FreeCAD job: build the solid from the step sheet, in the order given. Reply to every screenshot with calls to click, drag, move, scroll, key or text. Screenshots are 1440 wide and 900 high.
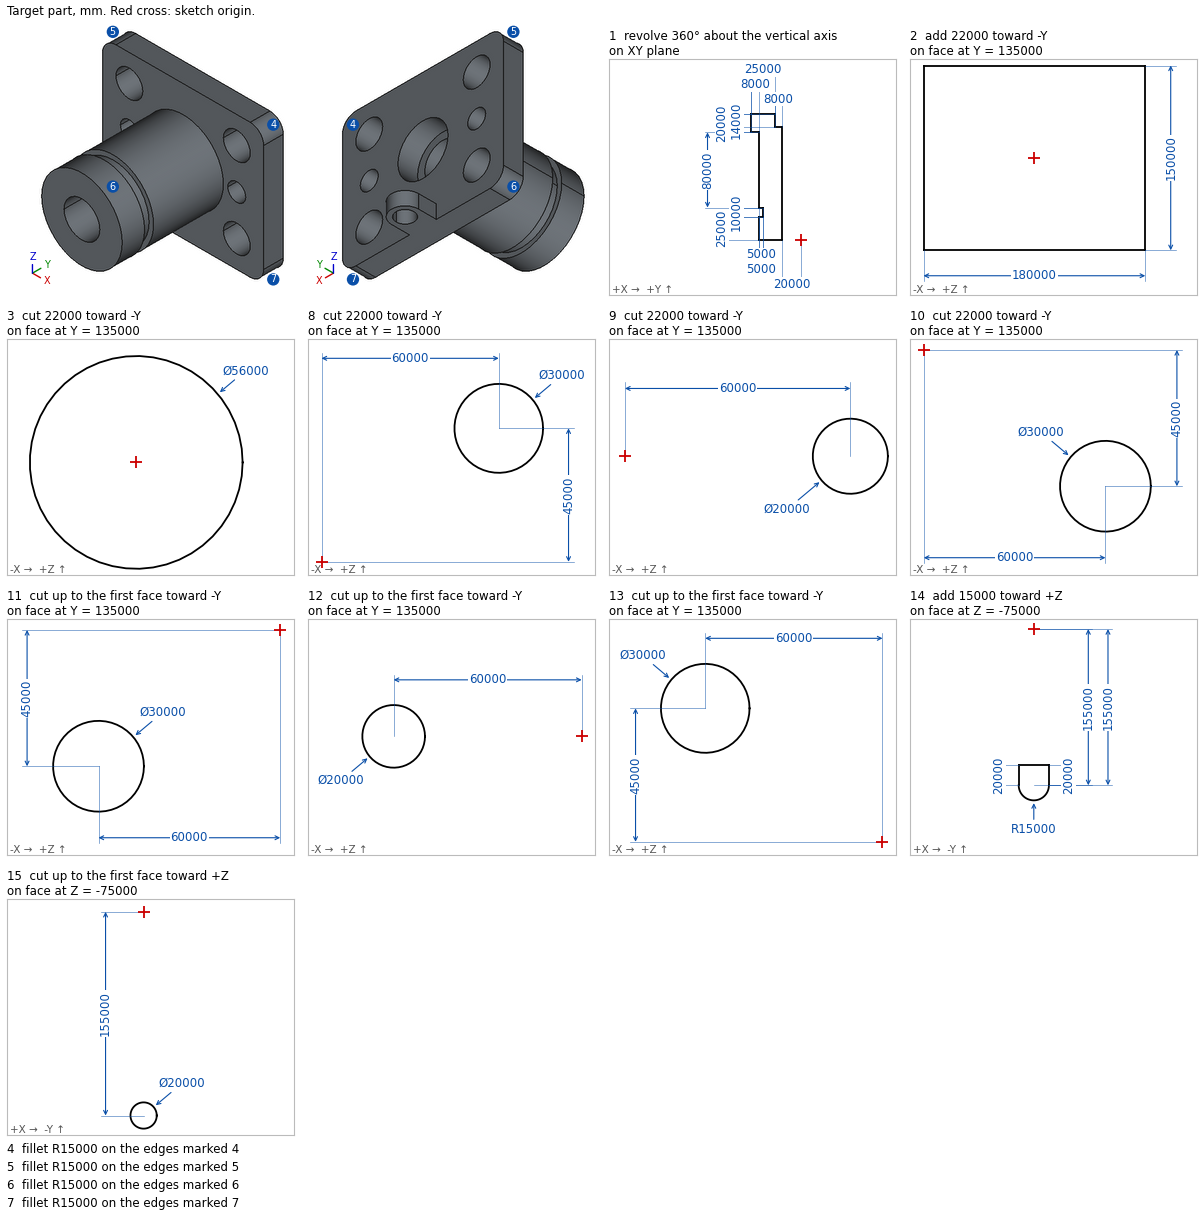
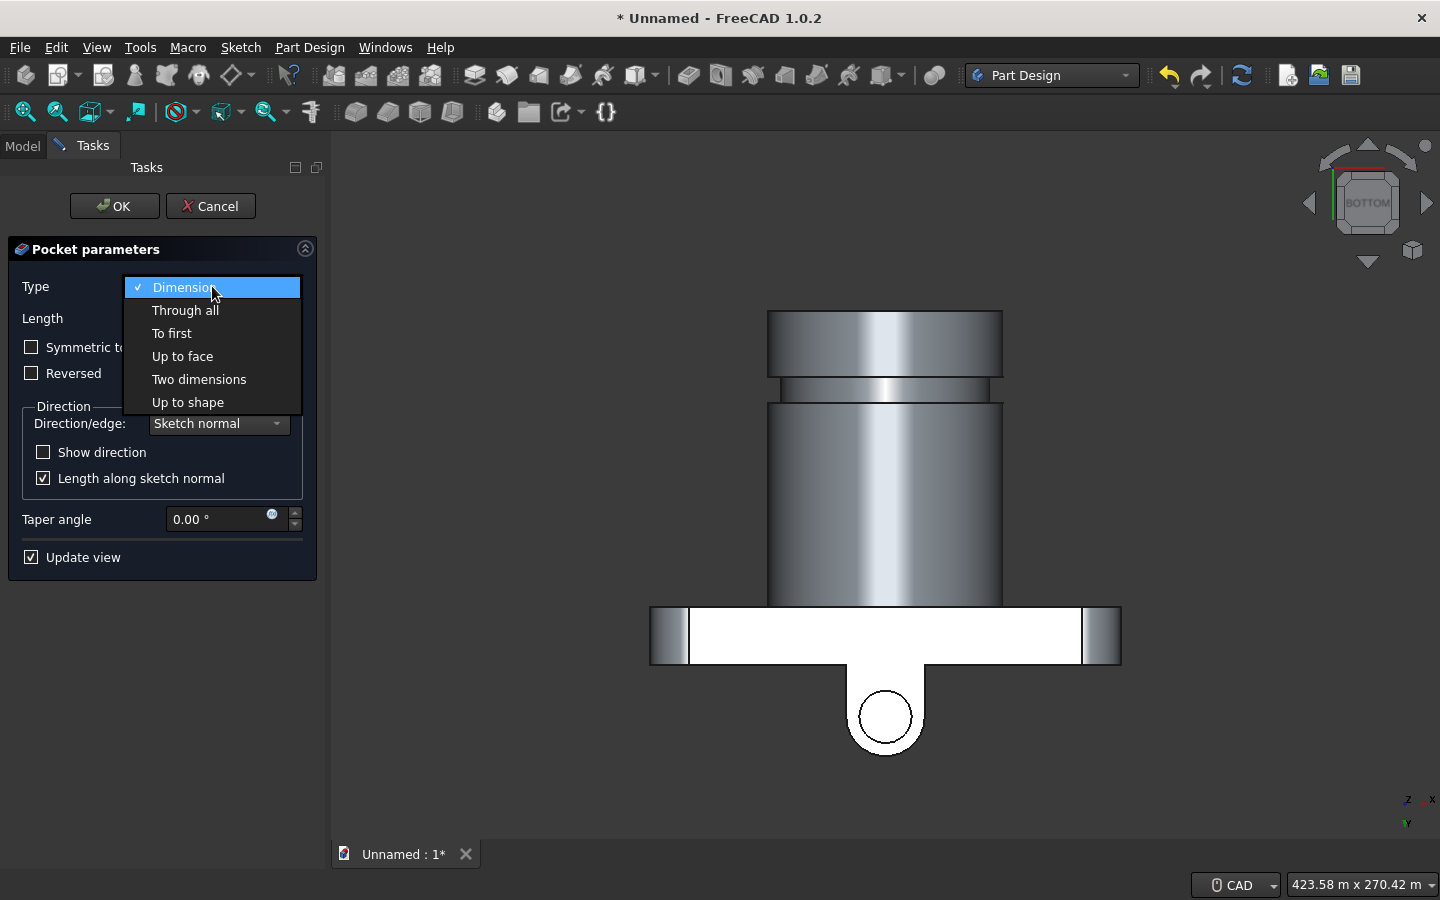
click(212, 334)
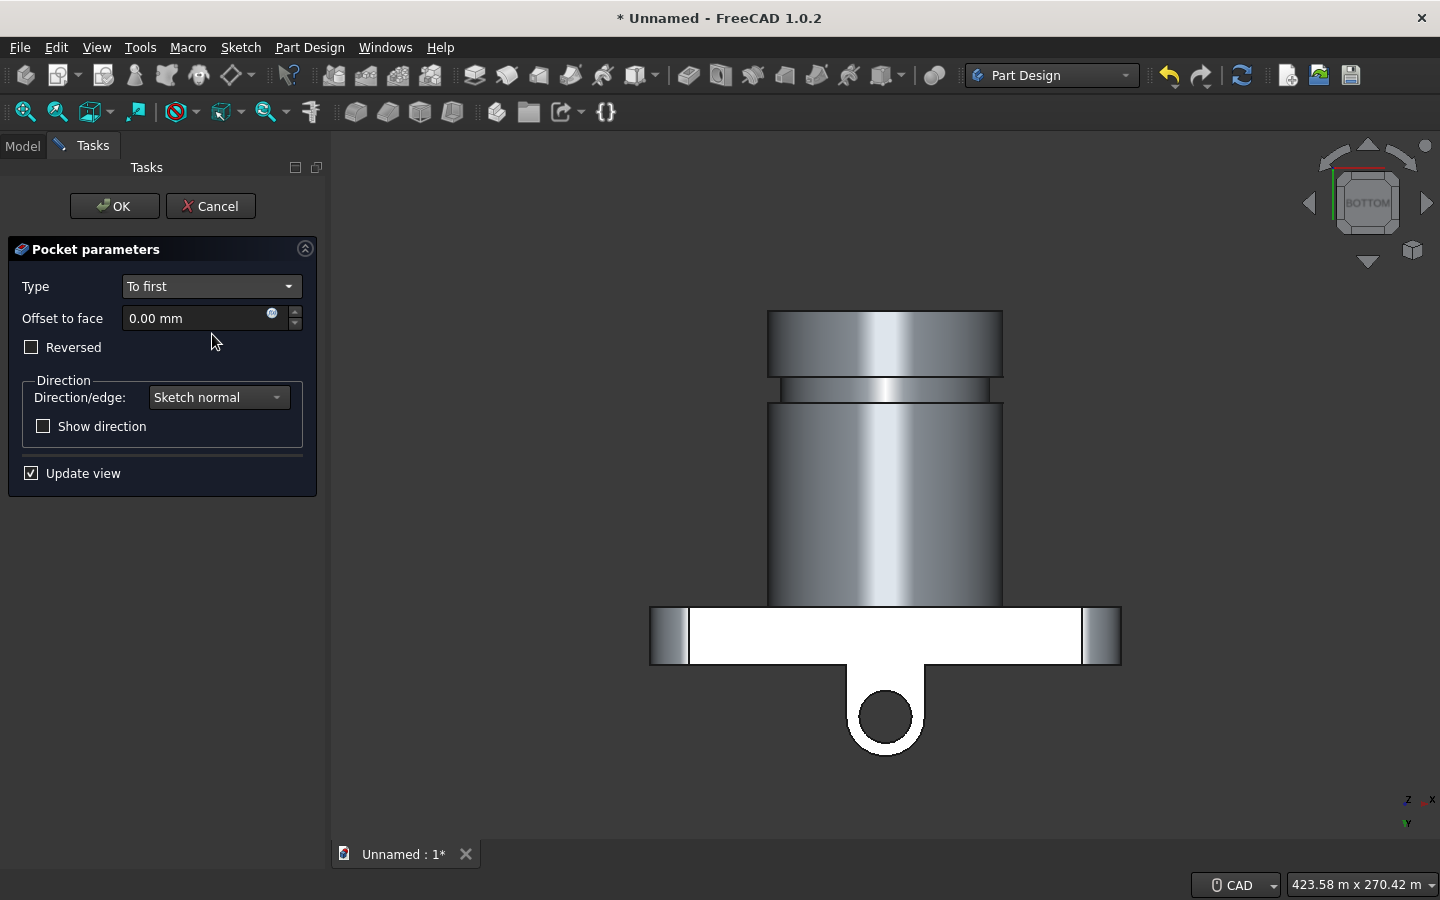
click(115, 206)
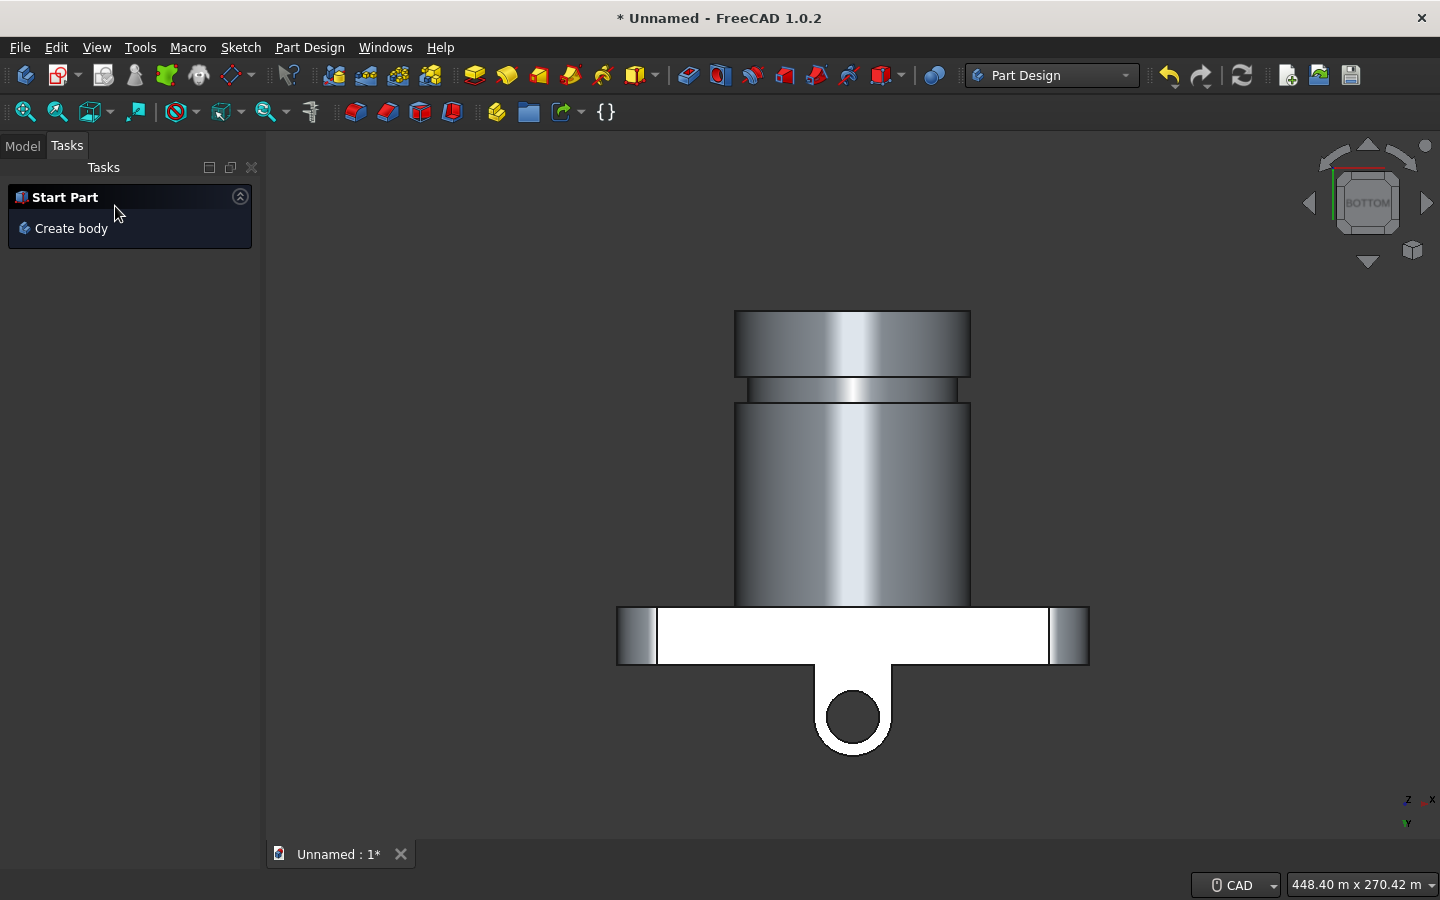
key(0)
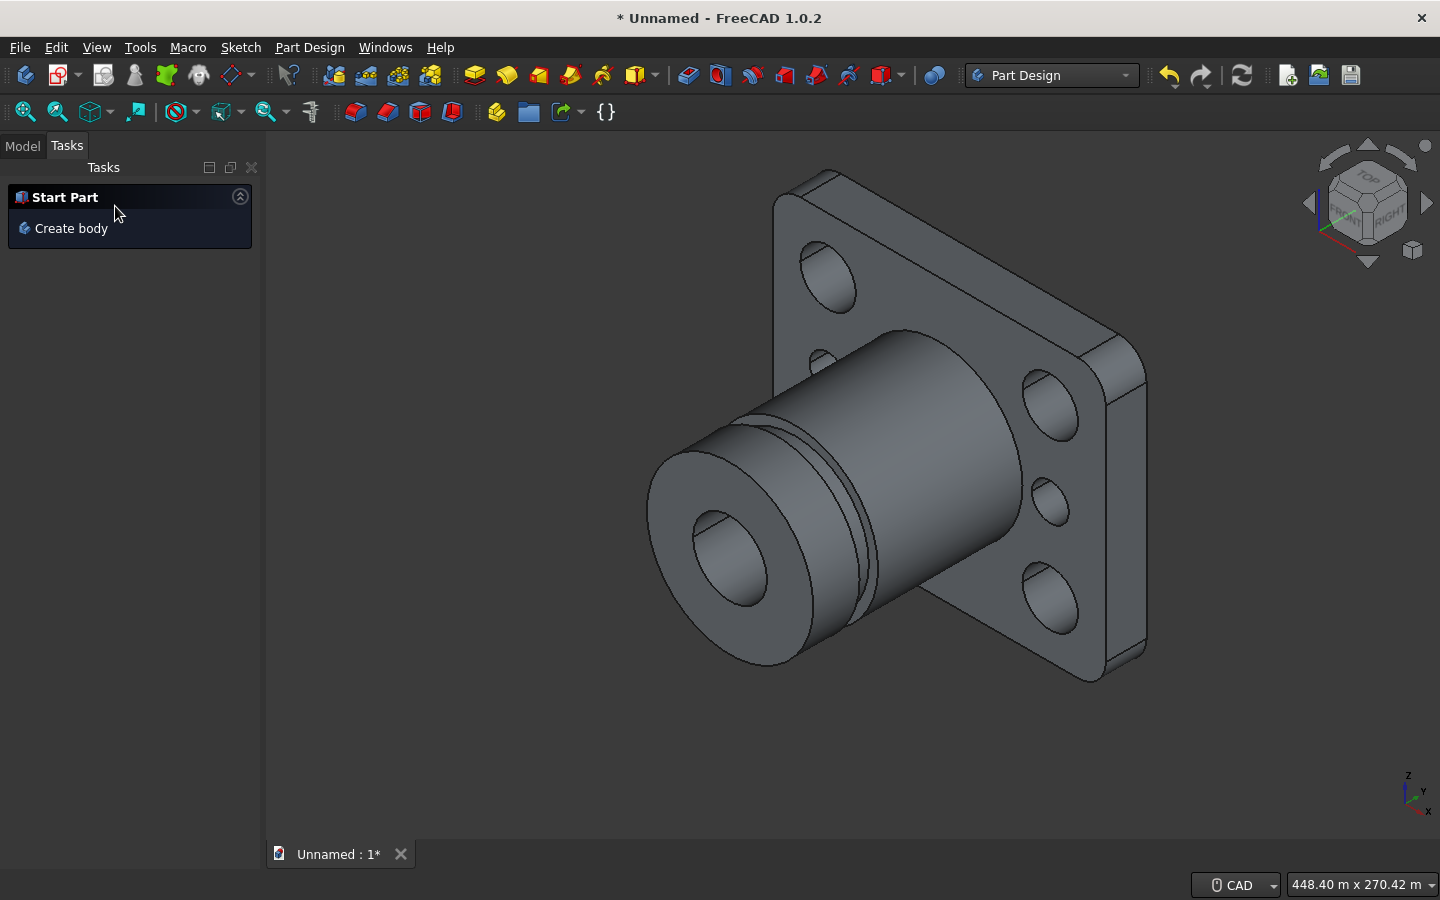
click(26, 112)